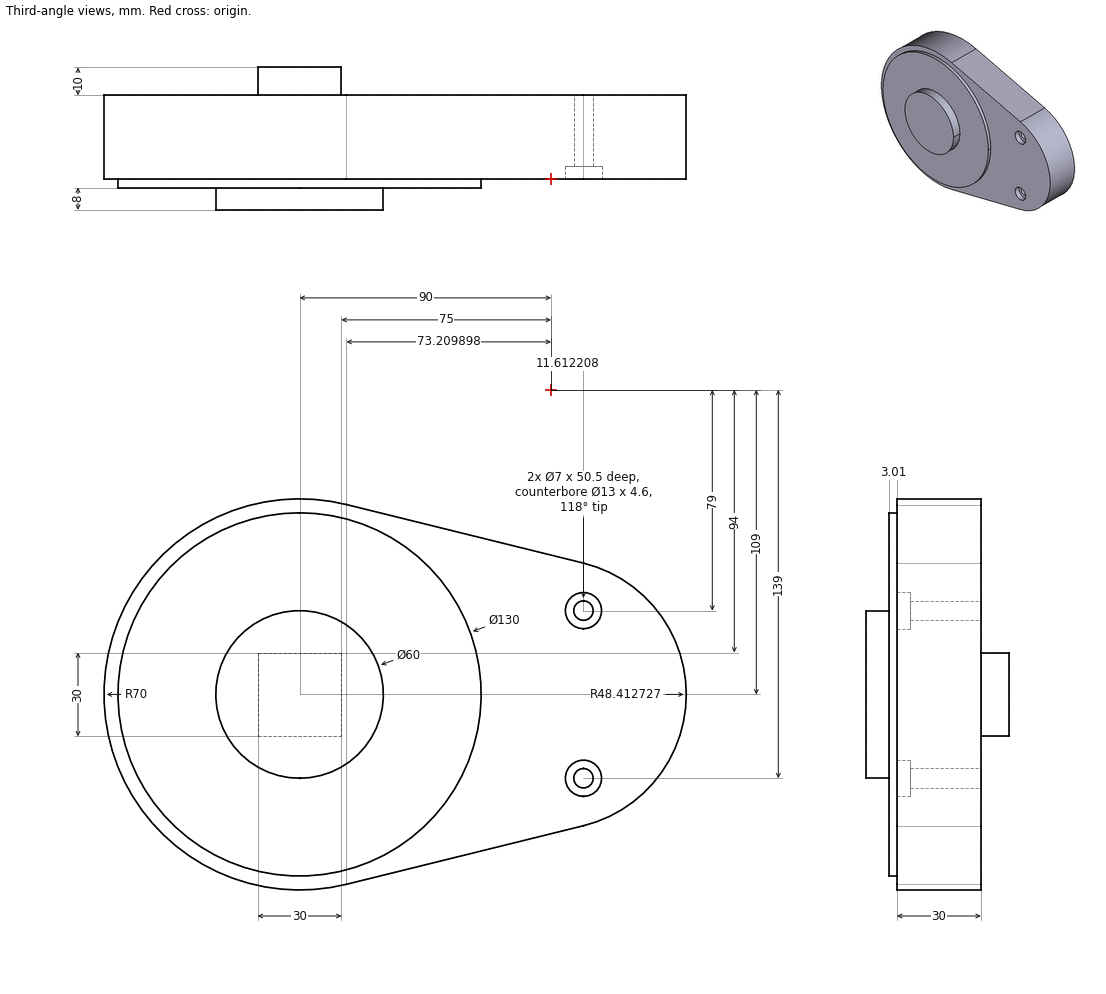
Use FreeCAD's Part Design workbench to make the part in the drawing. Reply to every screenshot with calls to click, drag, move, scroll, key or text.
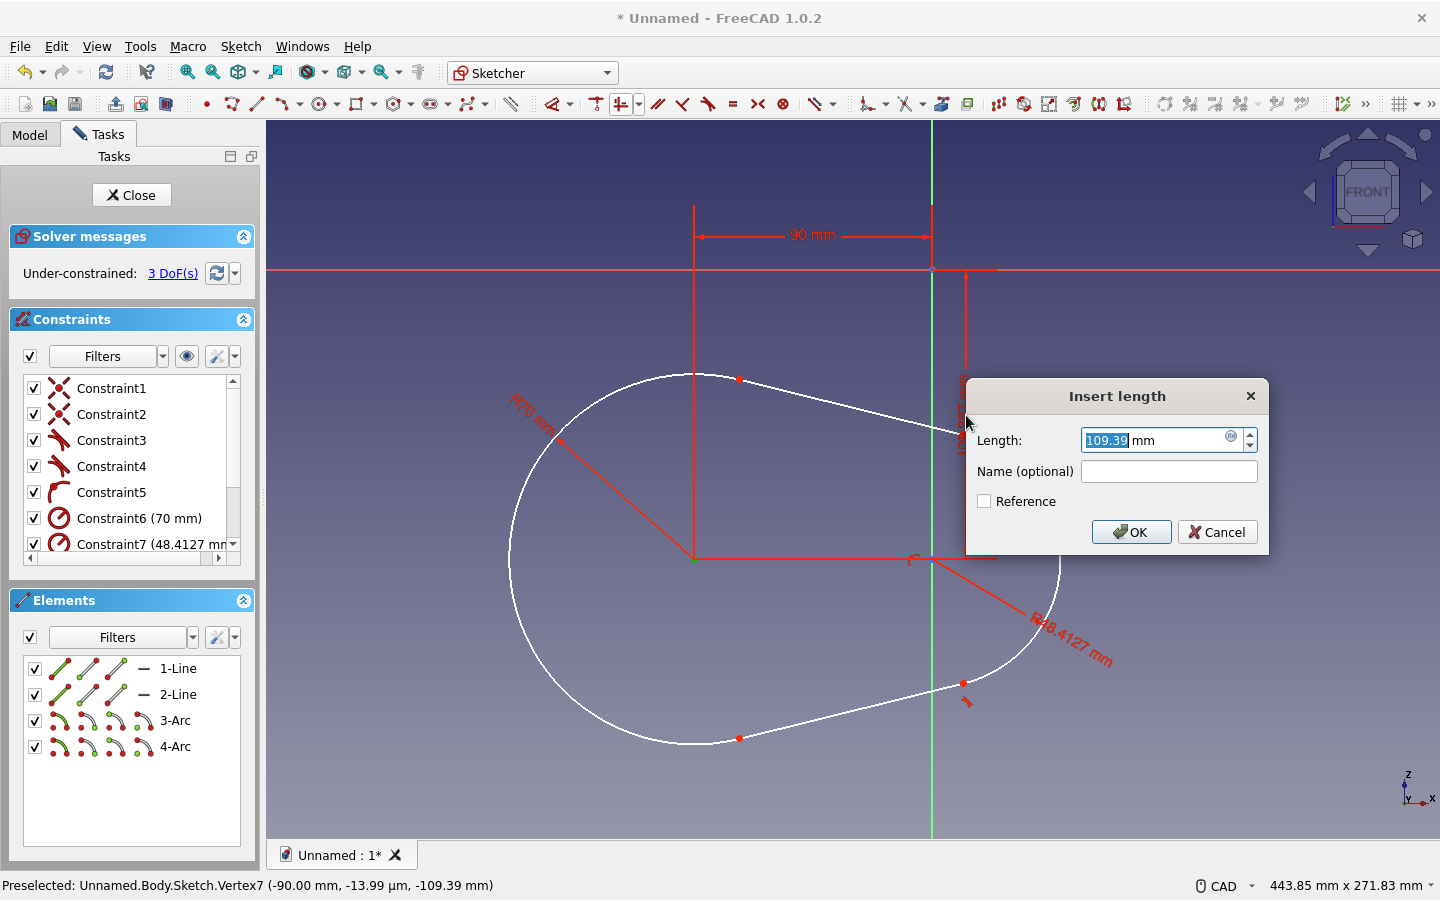
text(109)
key(Return)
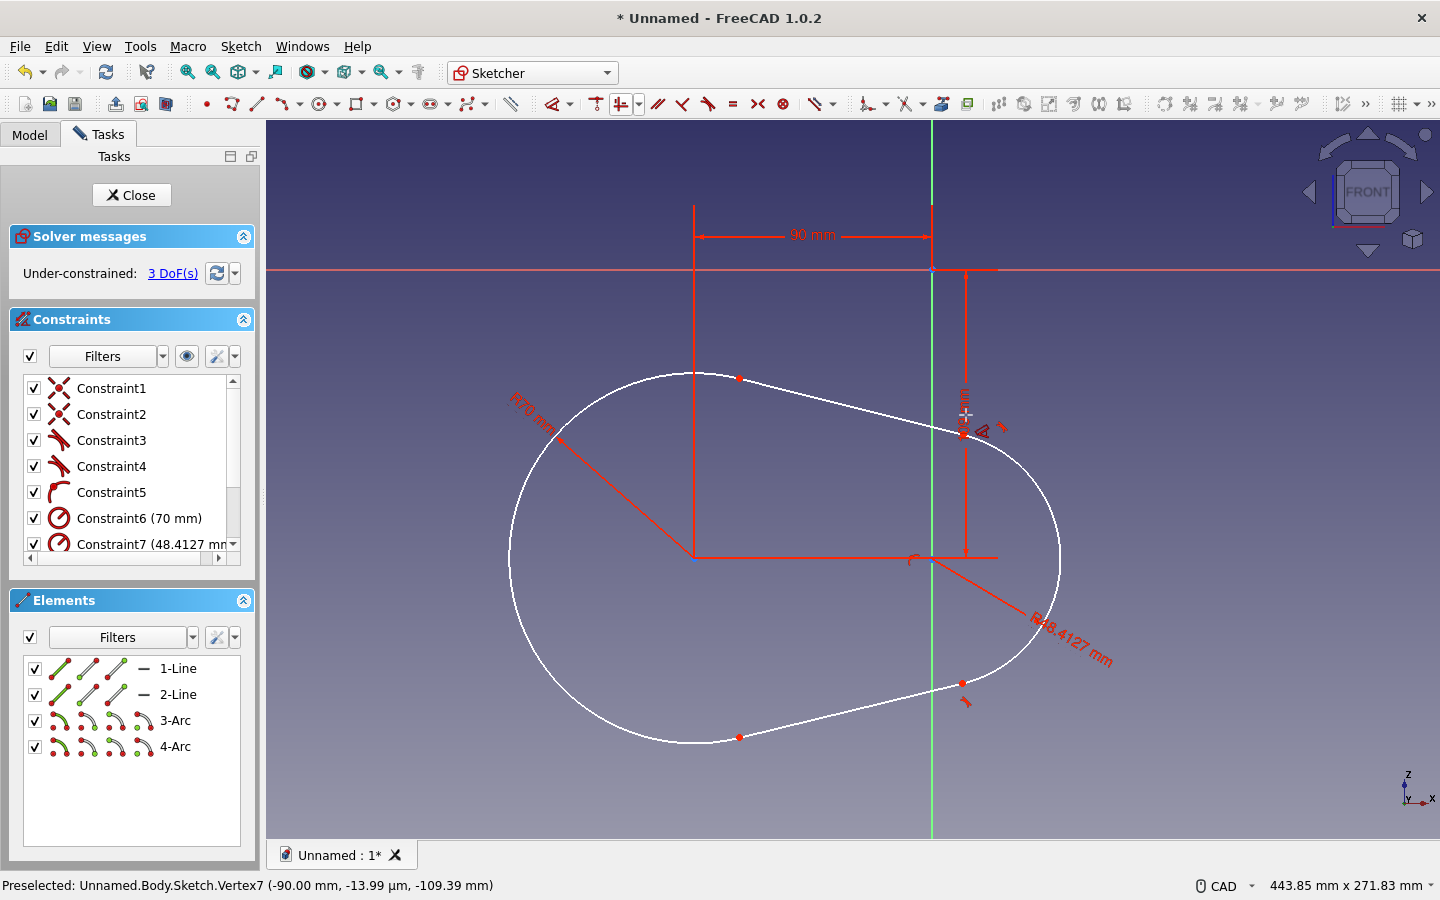
click(932, 559)
click(966, 348)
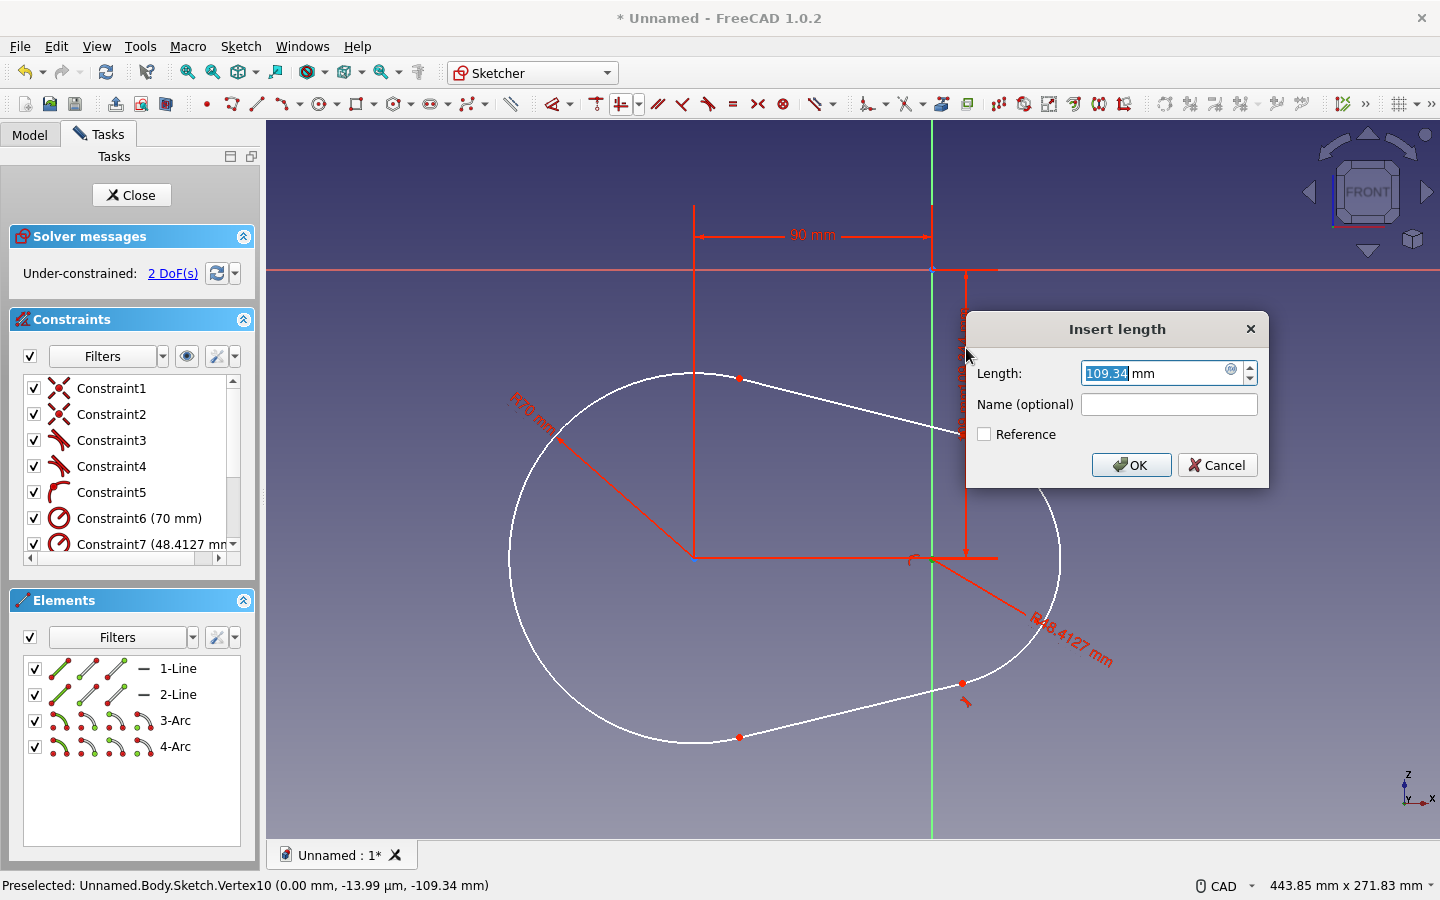
text(109)
key(Return)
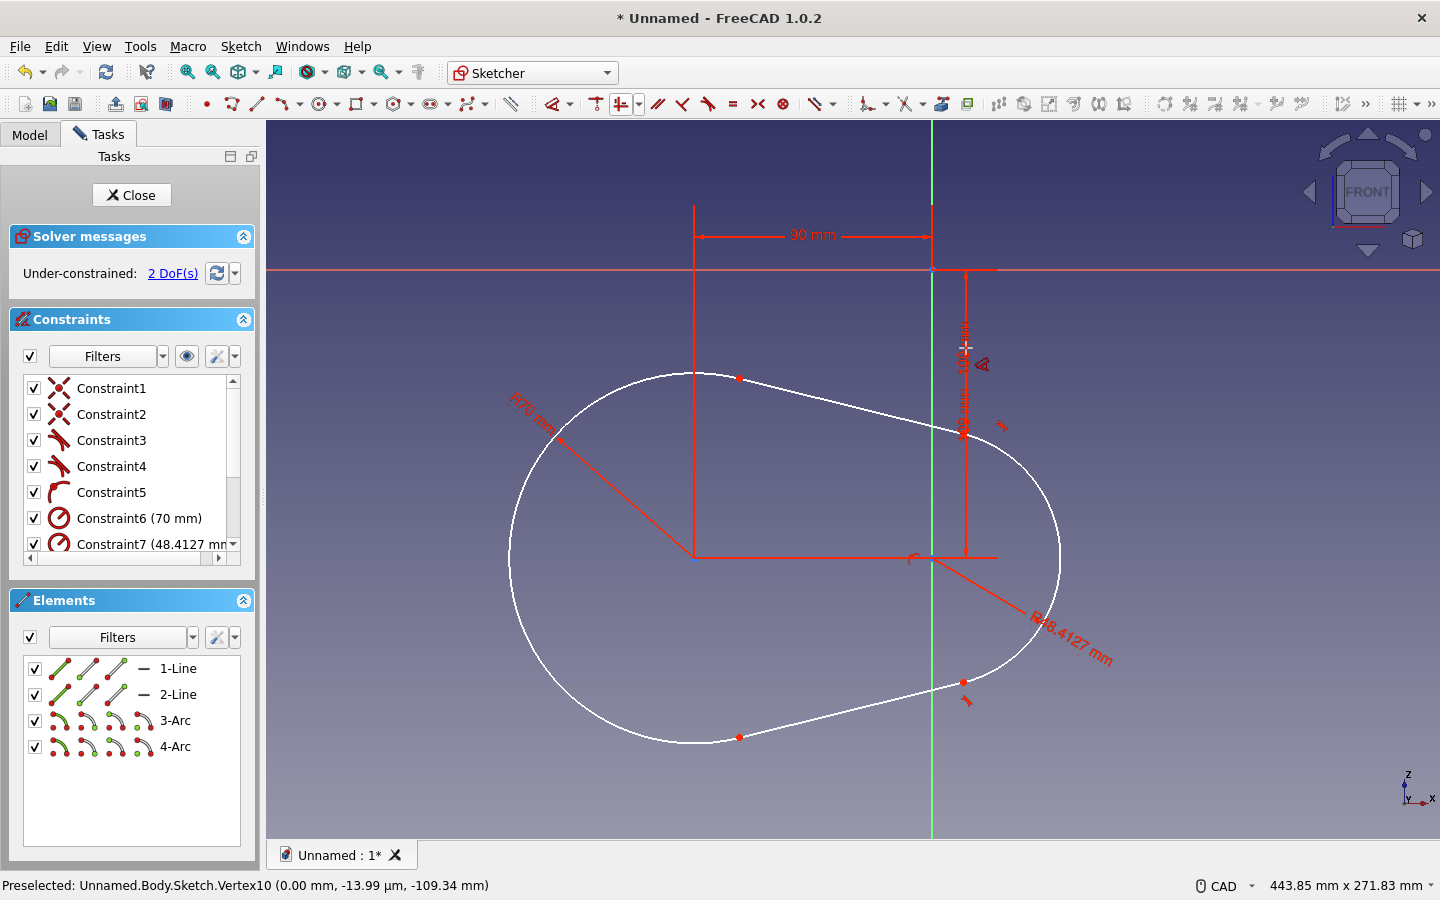
click(739, 738)
click(903, 236)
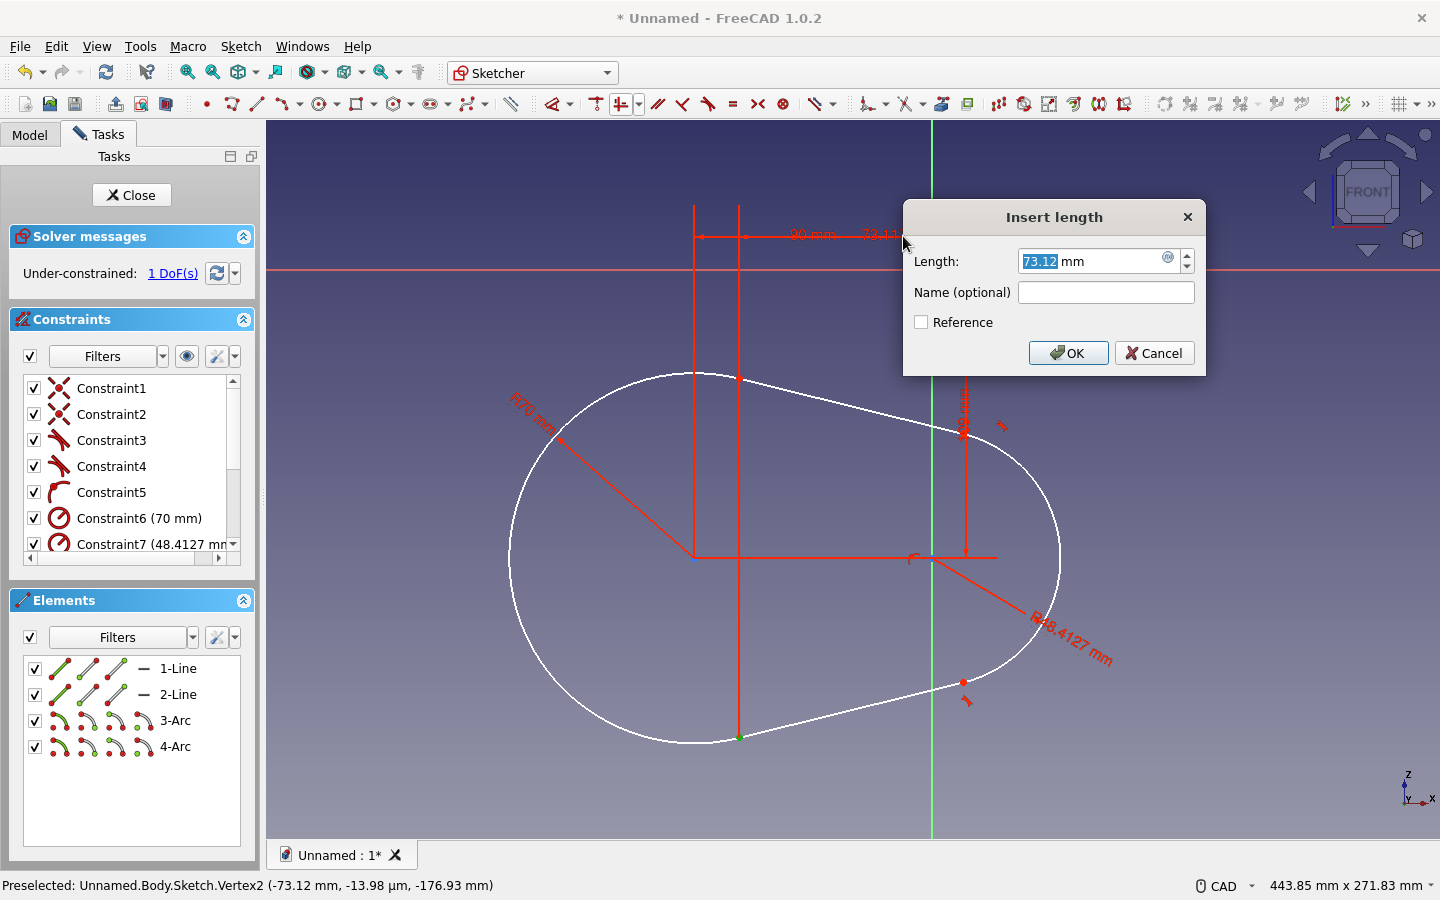
text(73.209898)
key(Return)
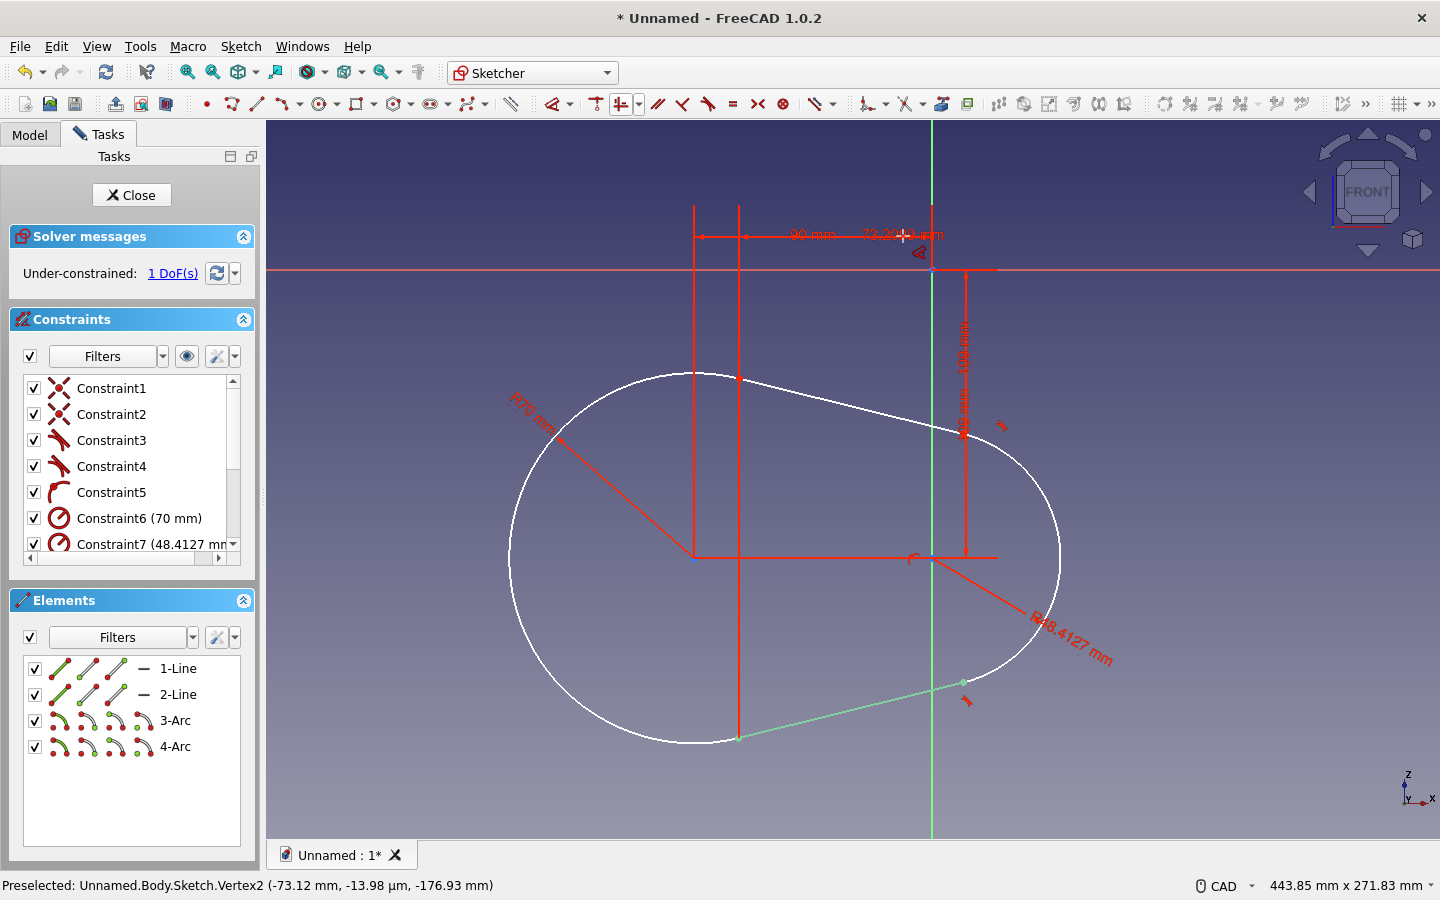
click(739, 379)
click(791, 413)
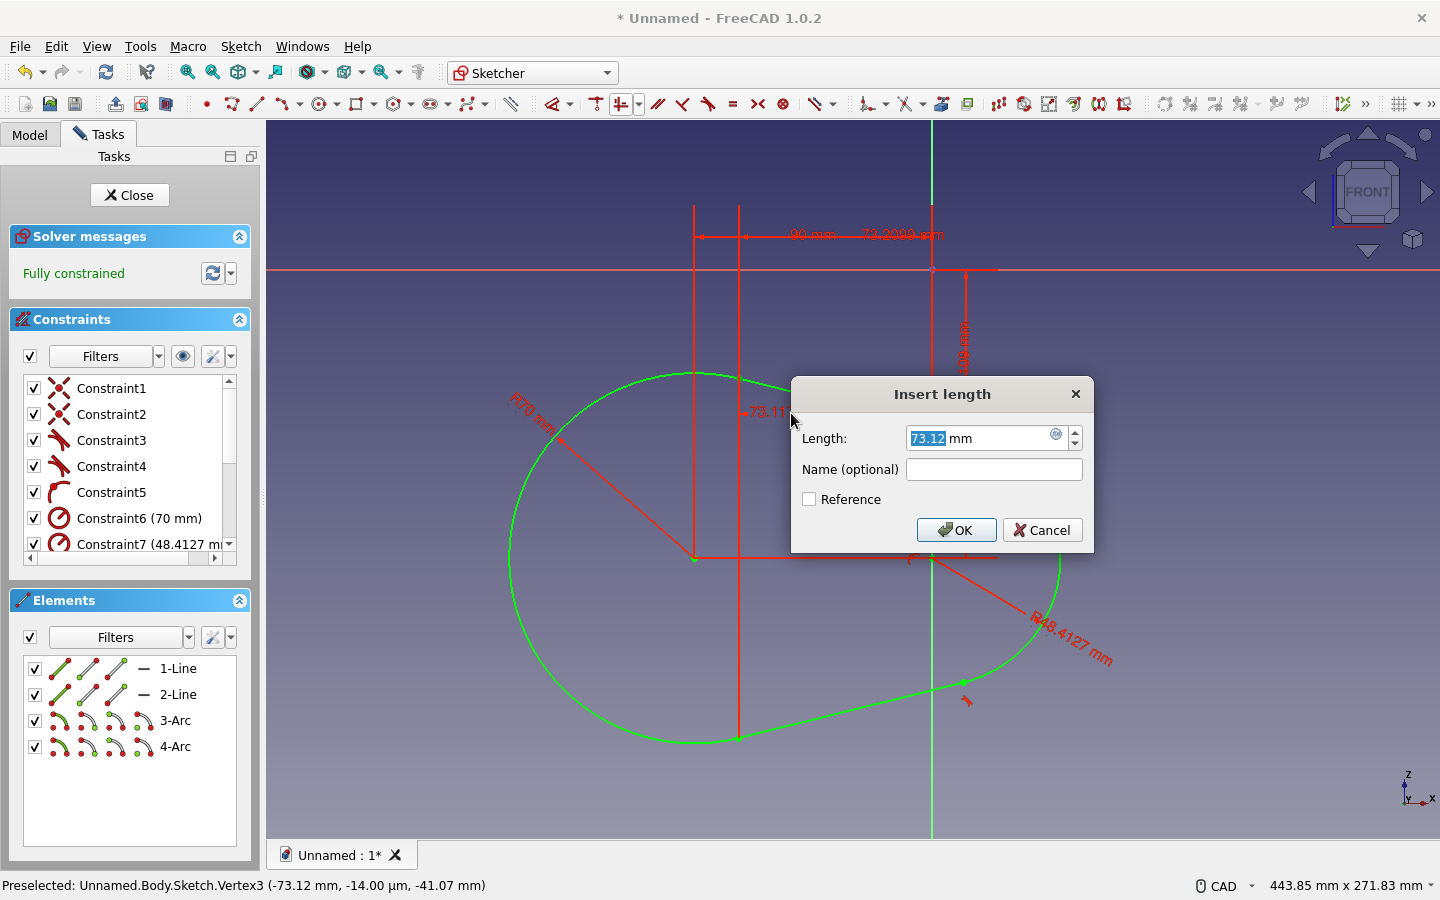
text(73.209898)
key(Return)
key(Escape)